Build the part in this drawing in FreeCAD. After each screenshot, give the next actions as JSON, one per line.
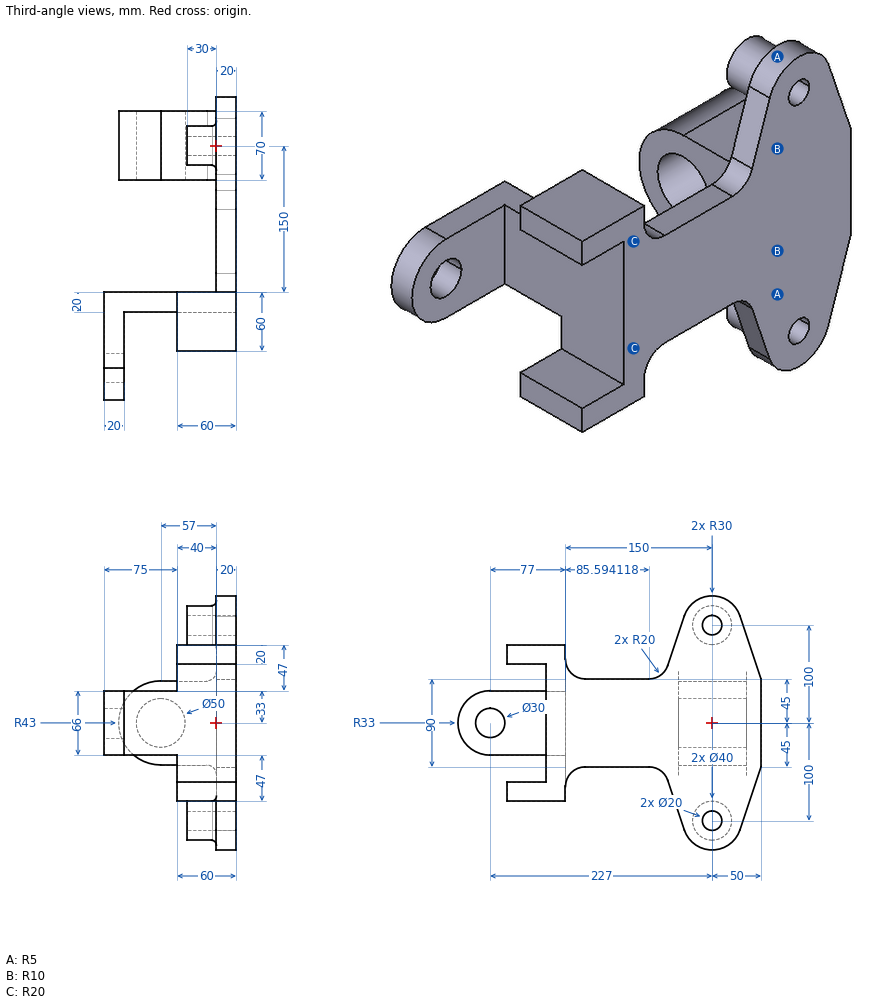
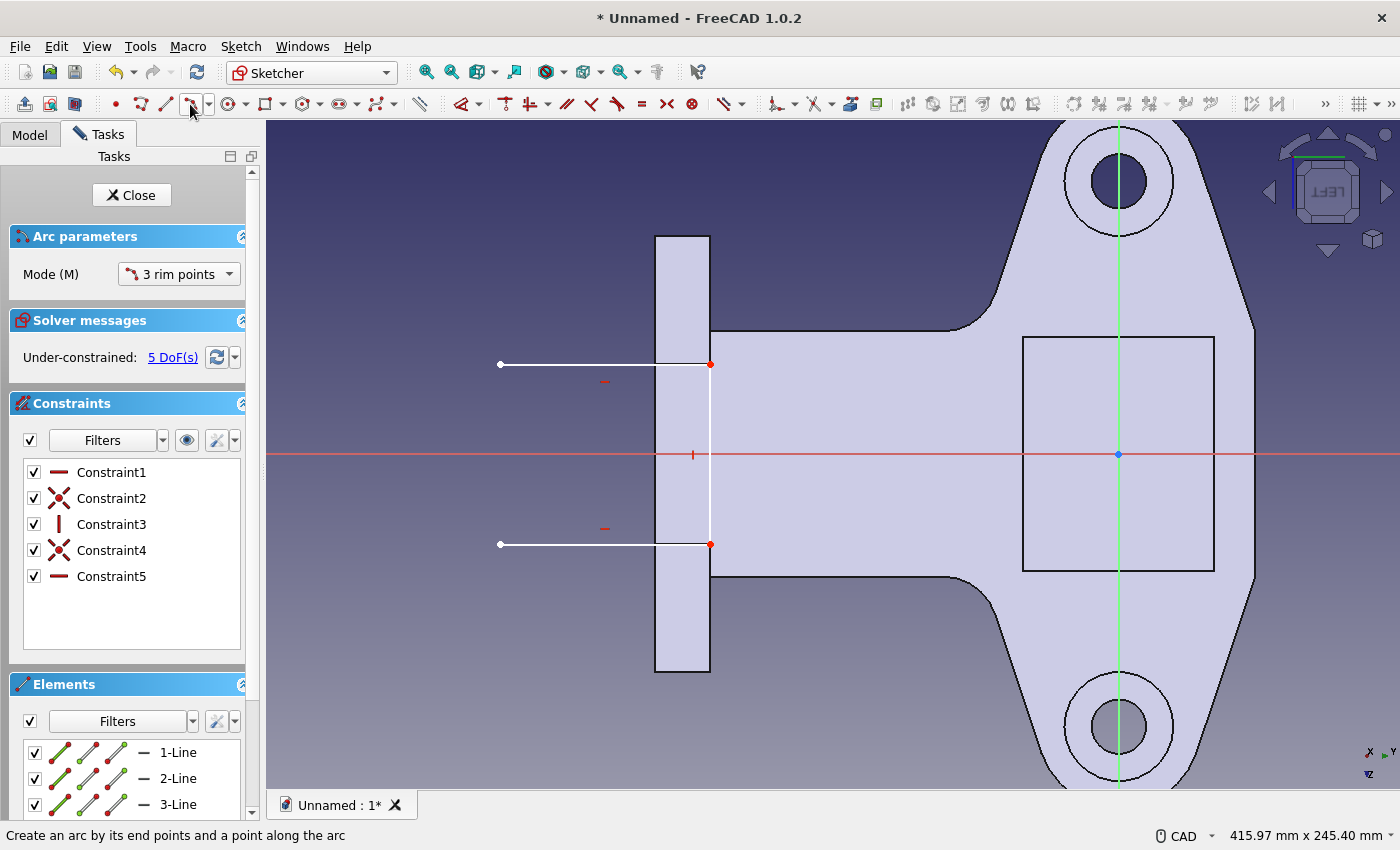
{"action": "left_click", "coordinate": [500, 365]}
{"action": "left_click", "coordinate": [500, 545]}
{"action": "left_click", "coordinate": [414, 426]}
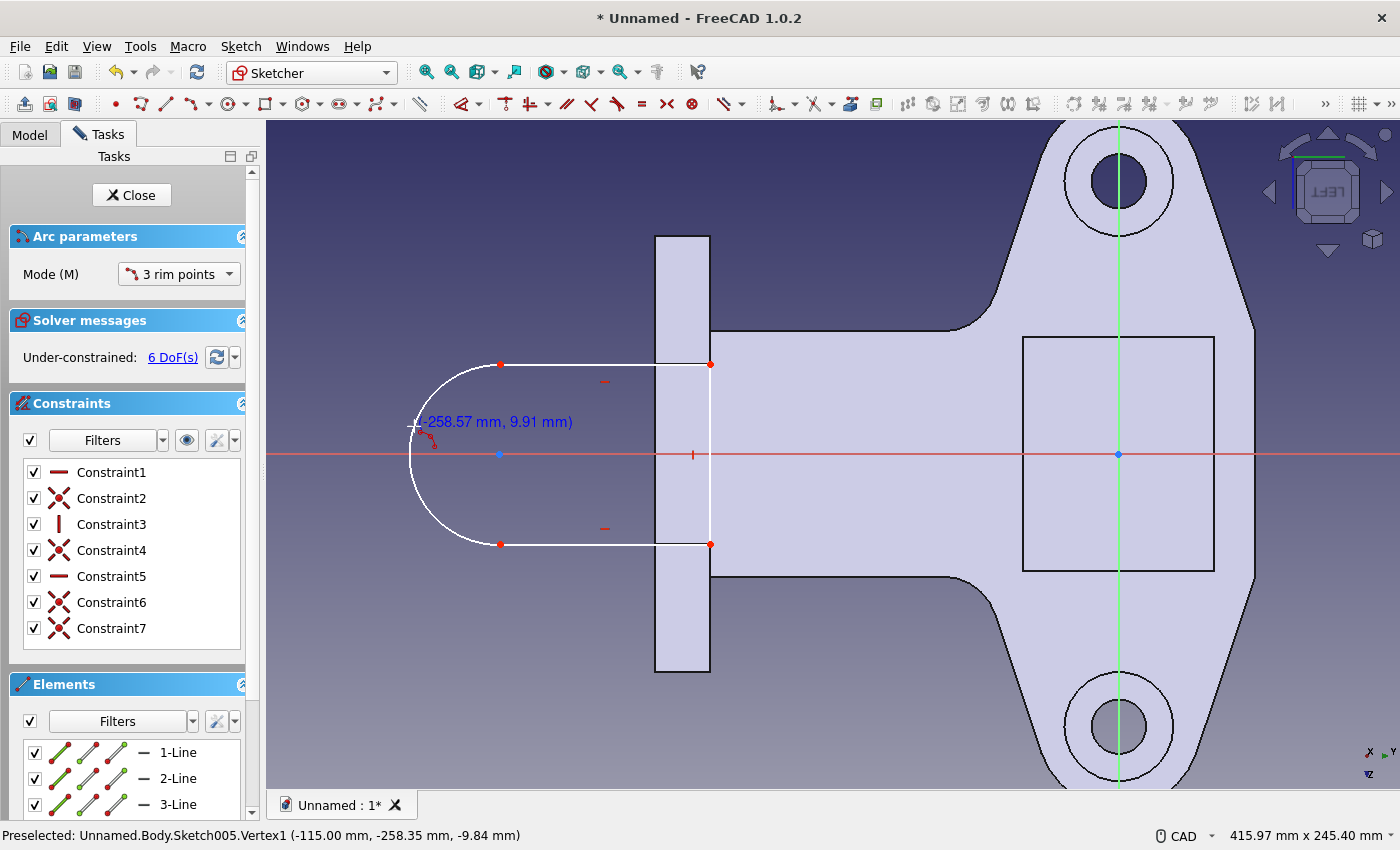
{"action": "left_click", "coordinate": [228, 104]}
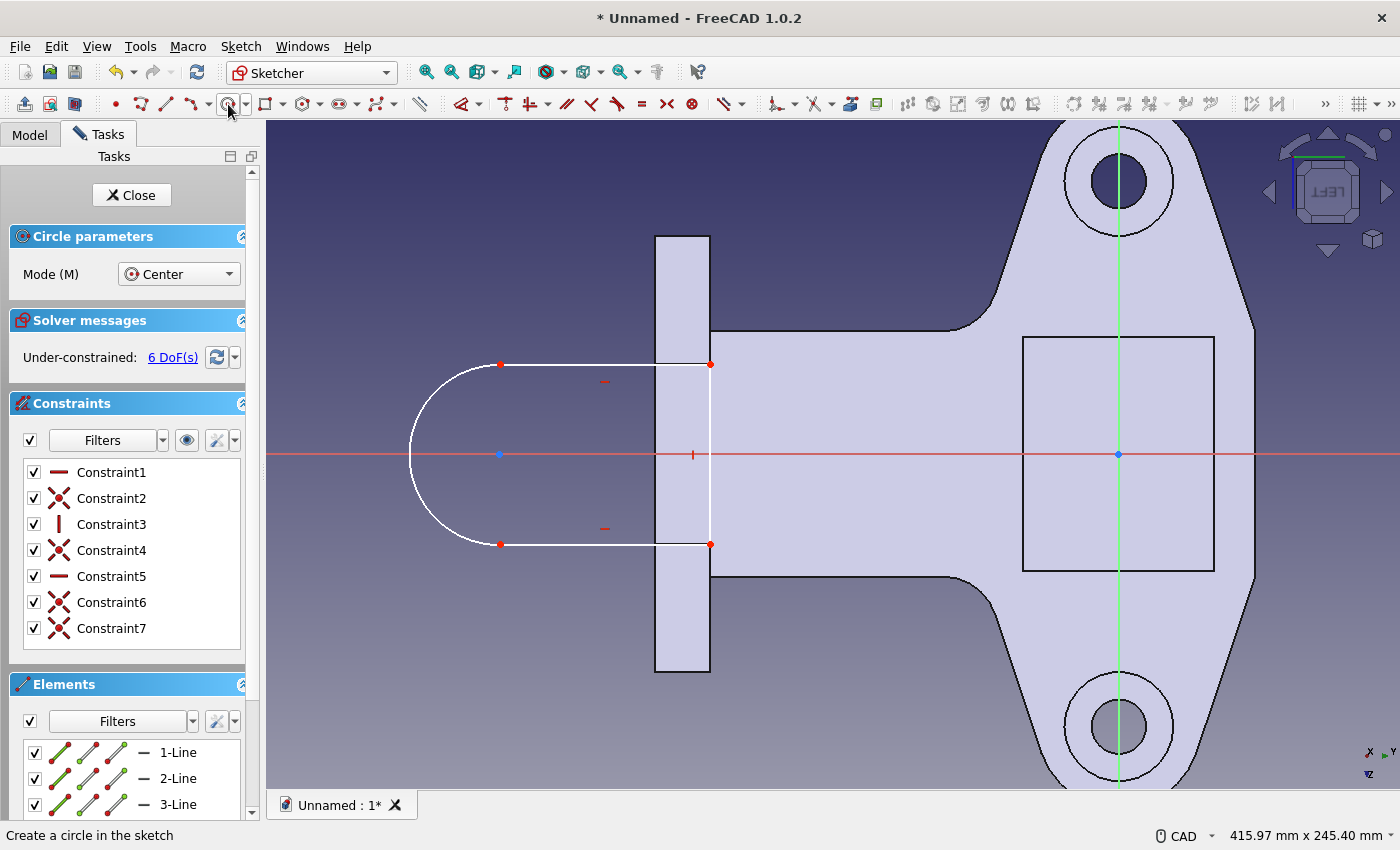
{"action": "left_click", "coordinate": [500, 454]}
{"action": "left_click", "coordinate": [529, 425]}
{"action": "key", "text": "Escape"}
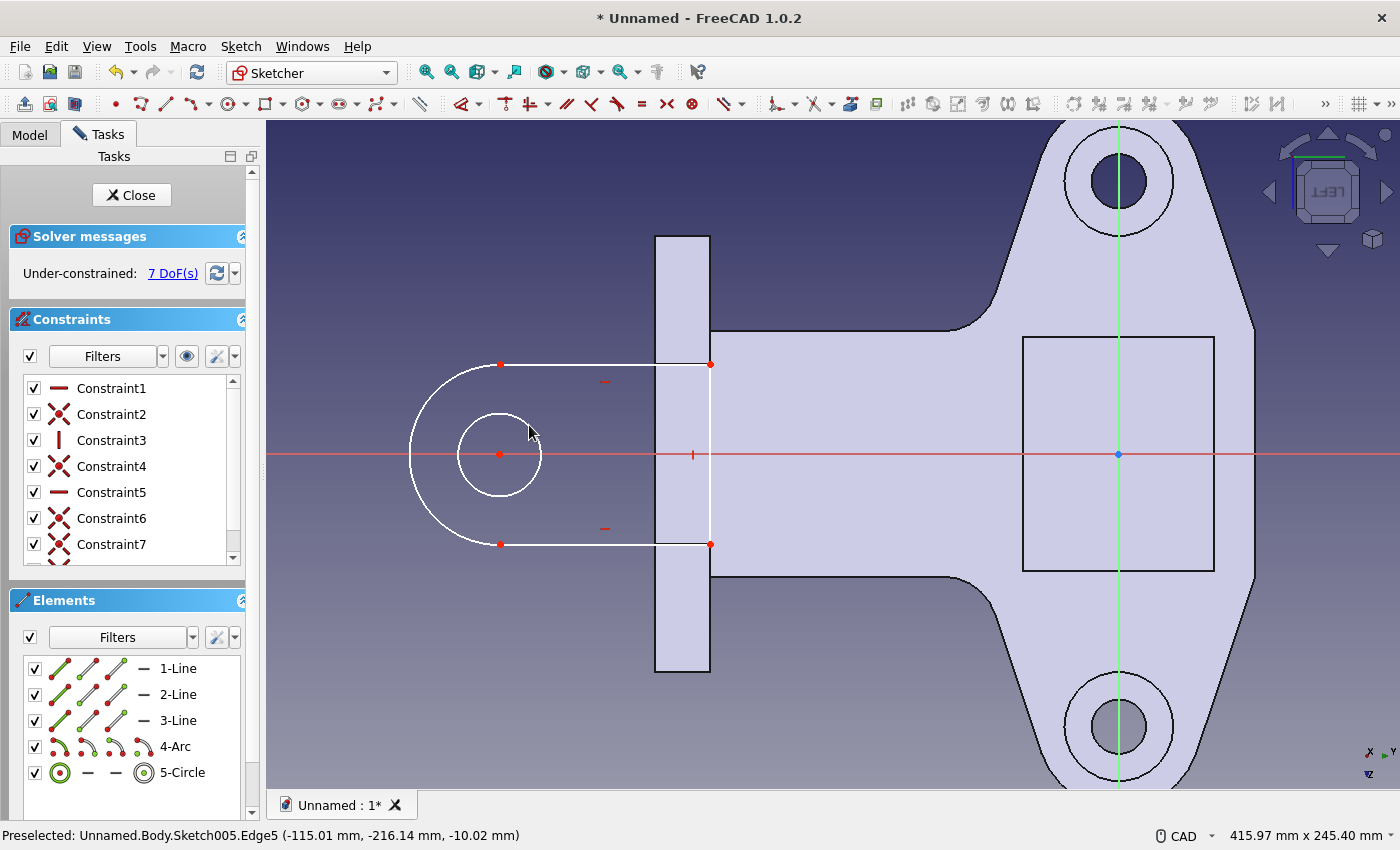
{"action": "left_click", "coordinate": [563, 545]}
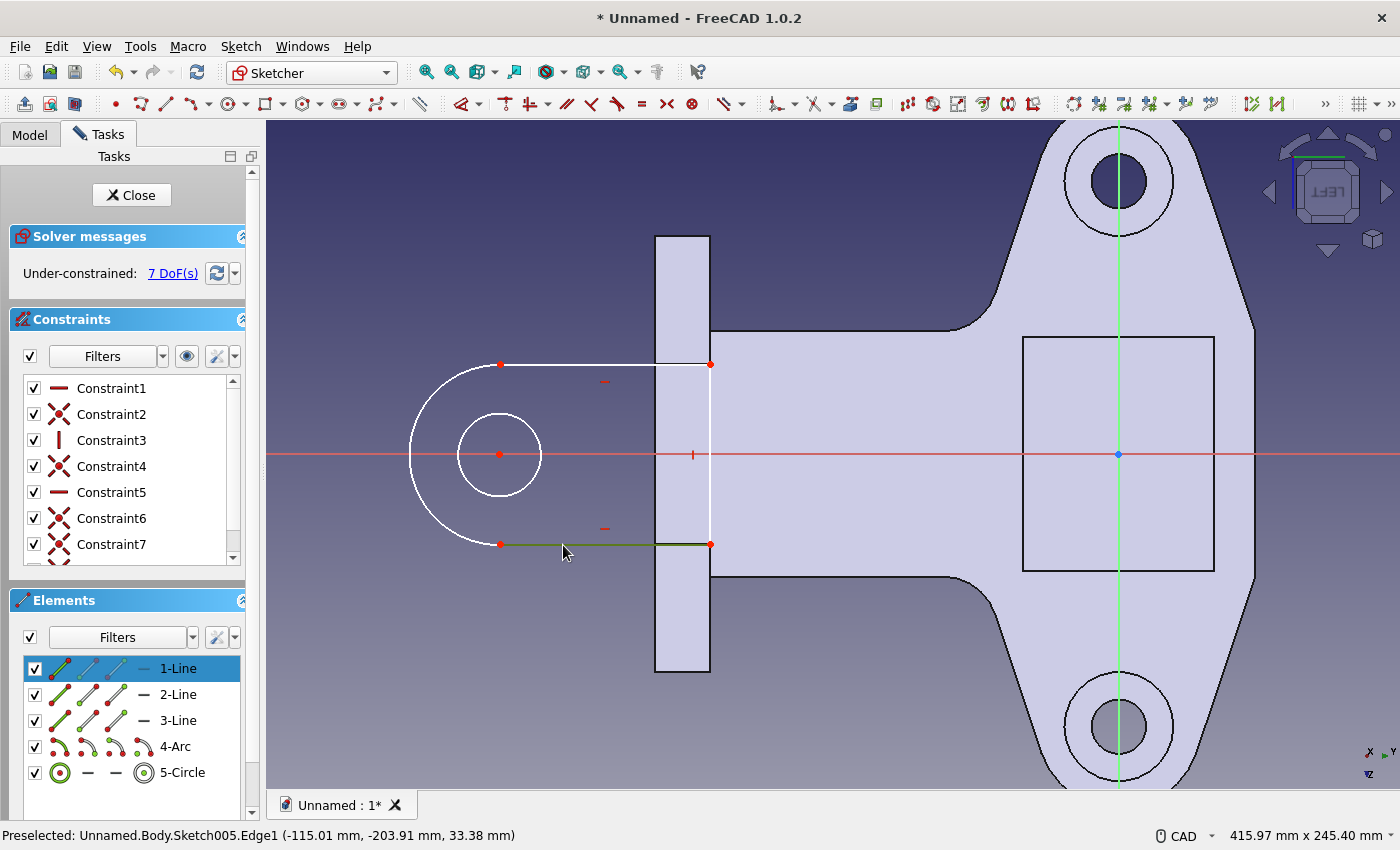
{"action": "left_click", "coordinate": [427, 402]}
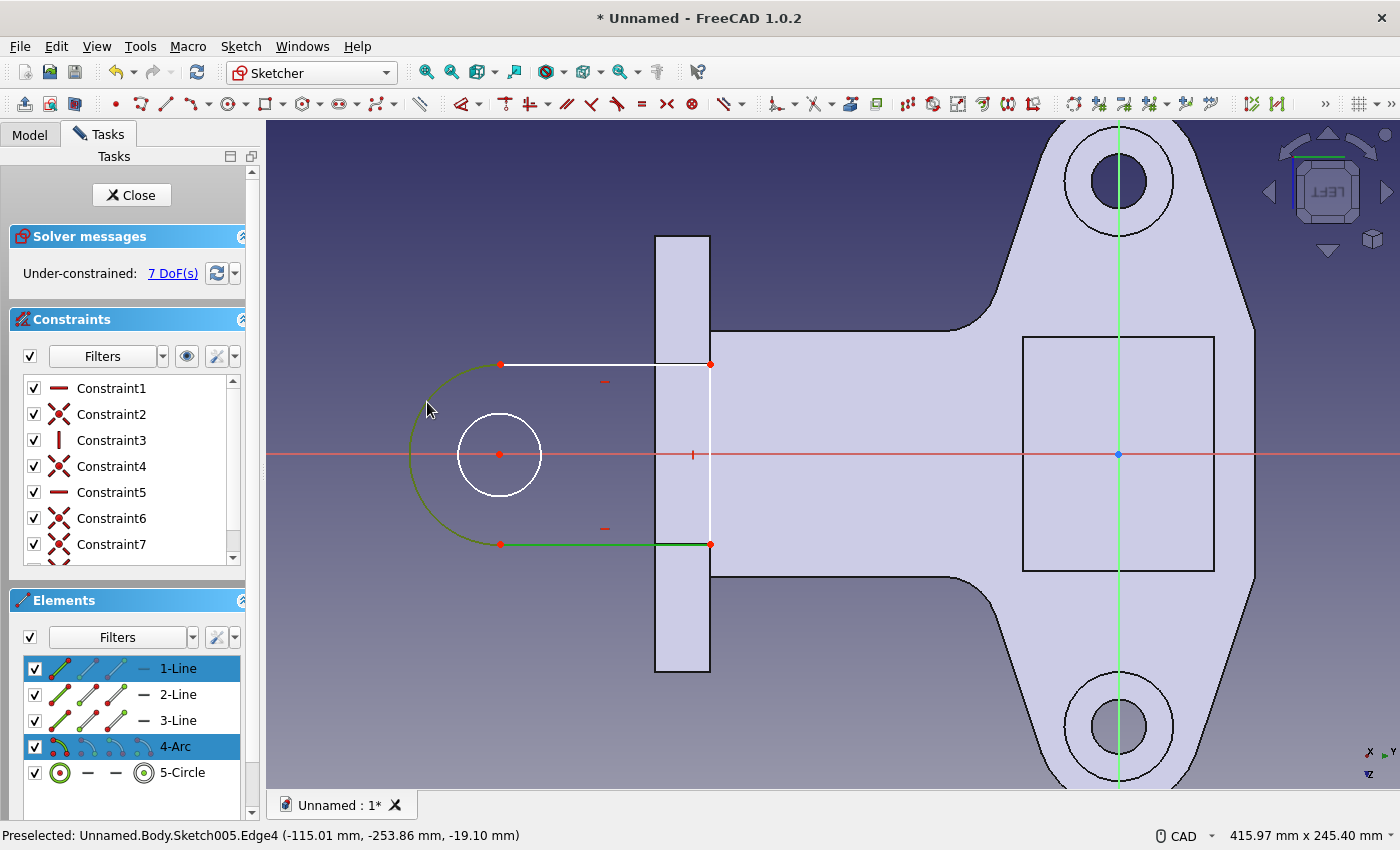
{"action": "key", "text": "t"}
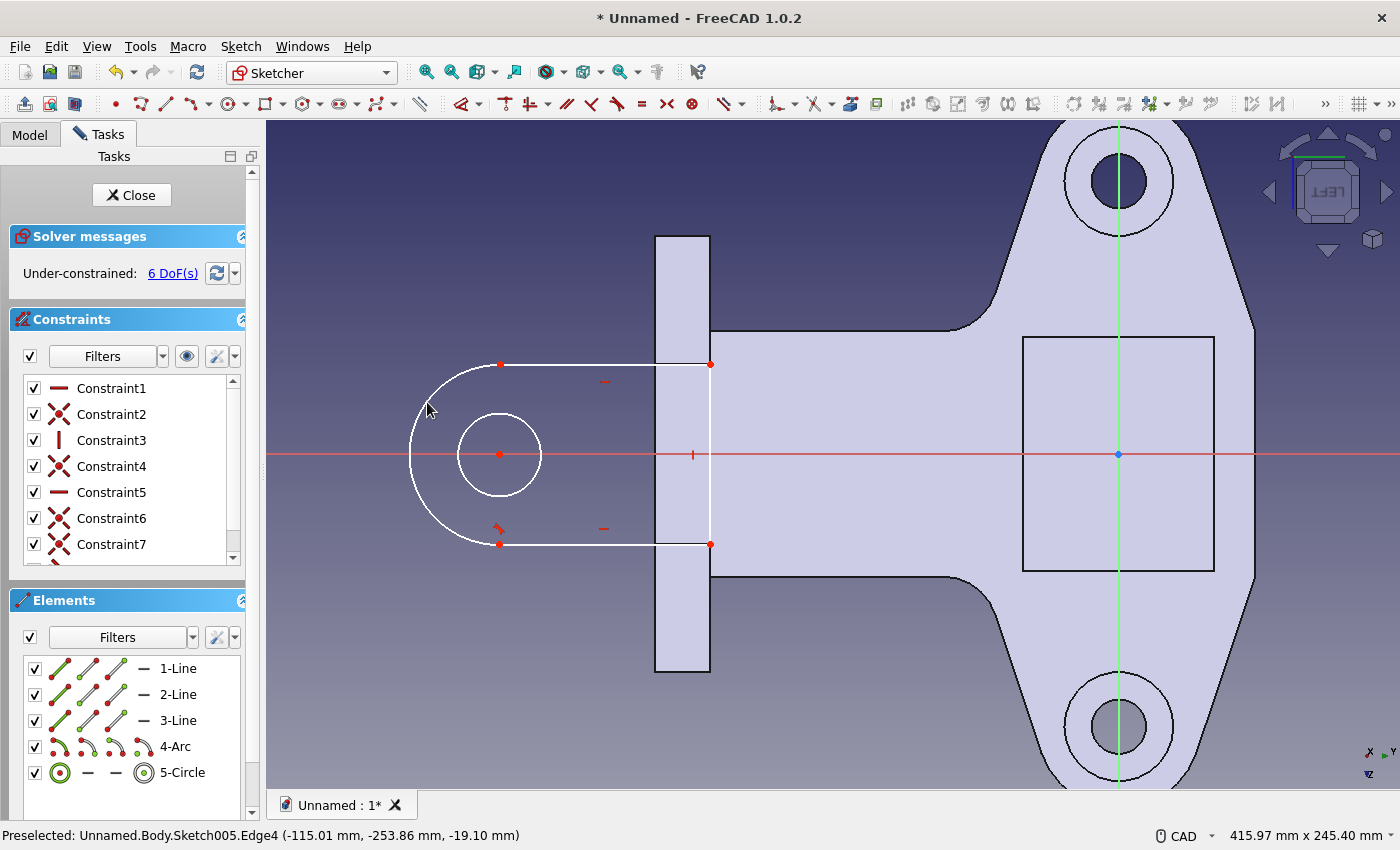
{"action": "left_click", "coordinate": [647, 365]}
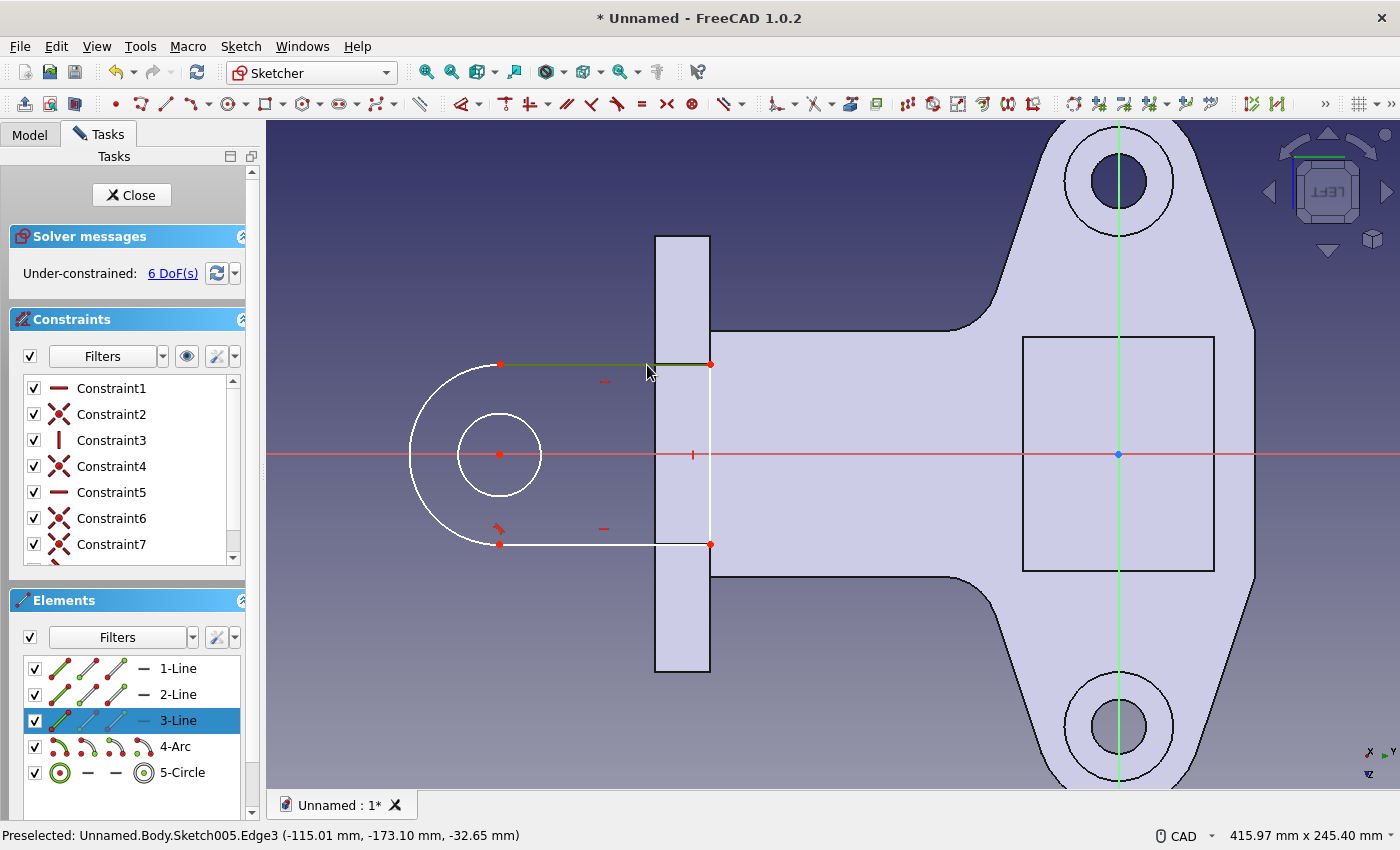
{"action": "left_click", "coordinate": [427, 402]}